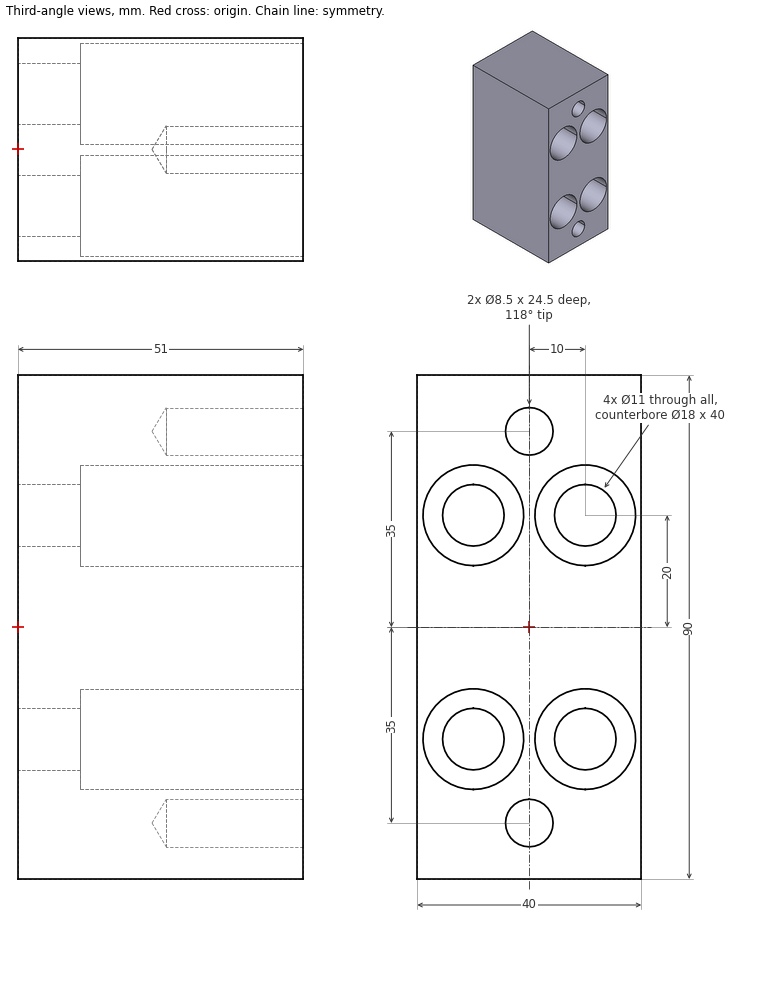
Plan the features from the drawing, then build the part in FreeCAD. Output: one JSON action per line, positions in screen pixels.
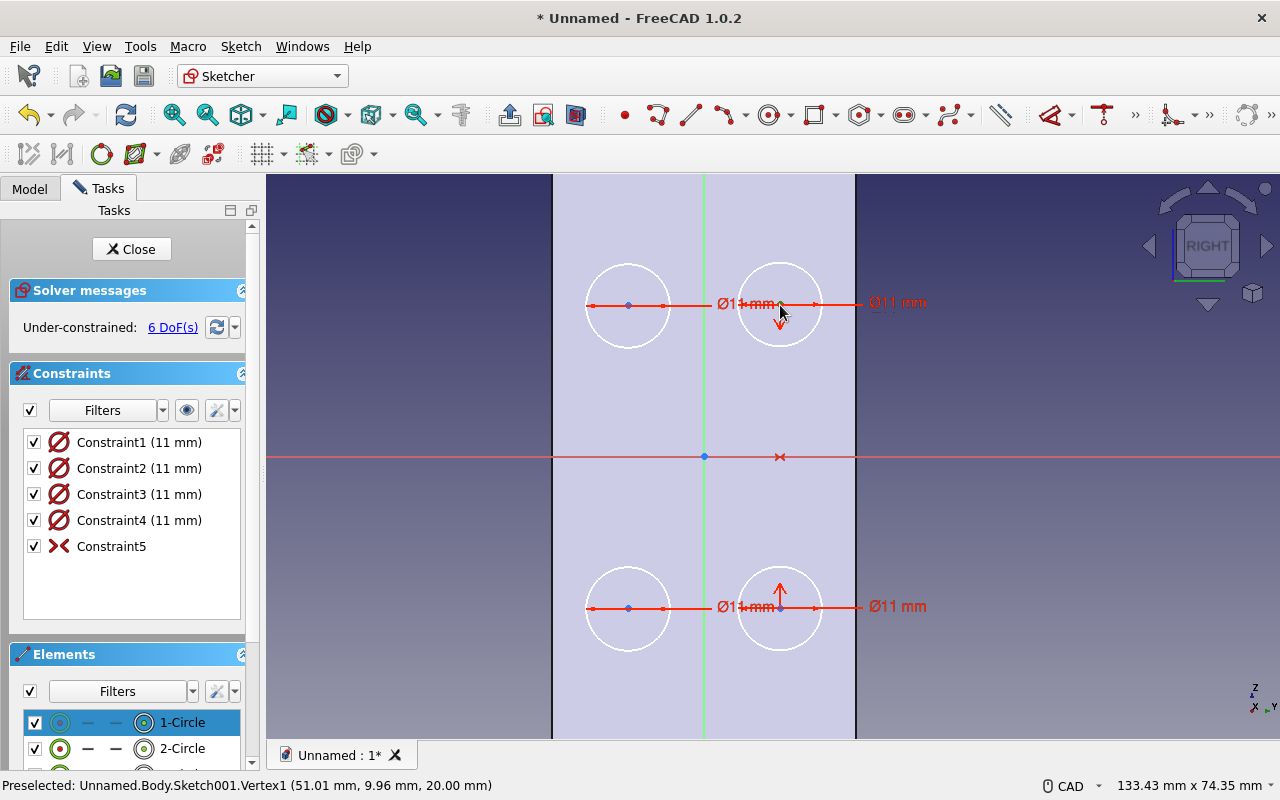
{"action": "left_click", "coordinate": [628, 306]}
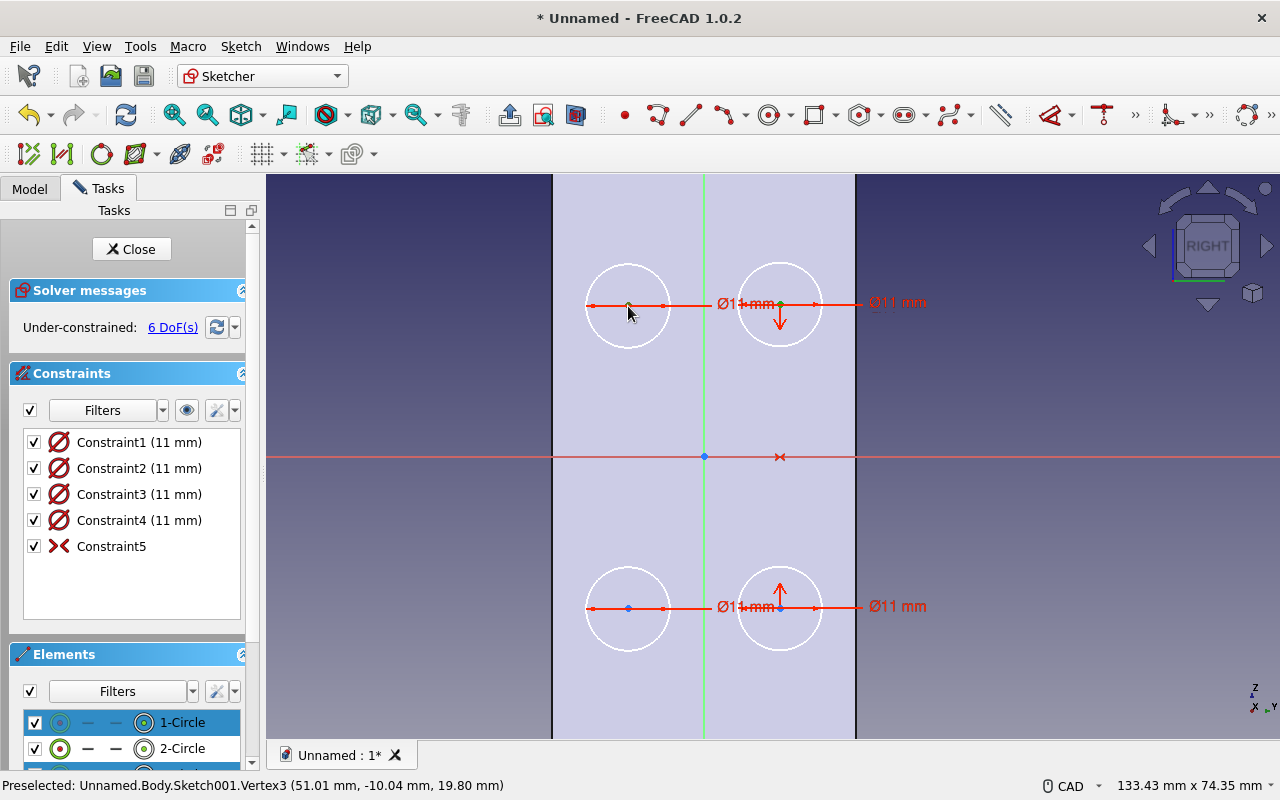
{"action": "left_click", "coordinate": [704, 675]}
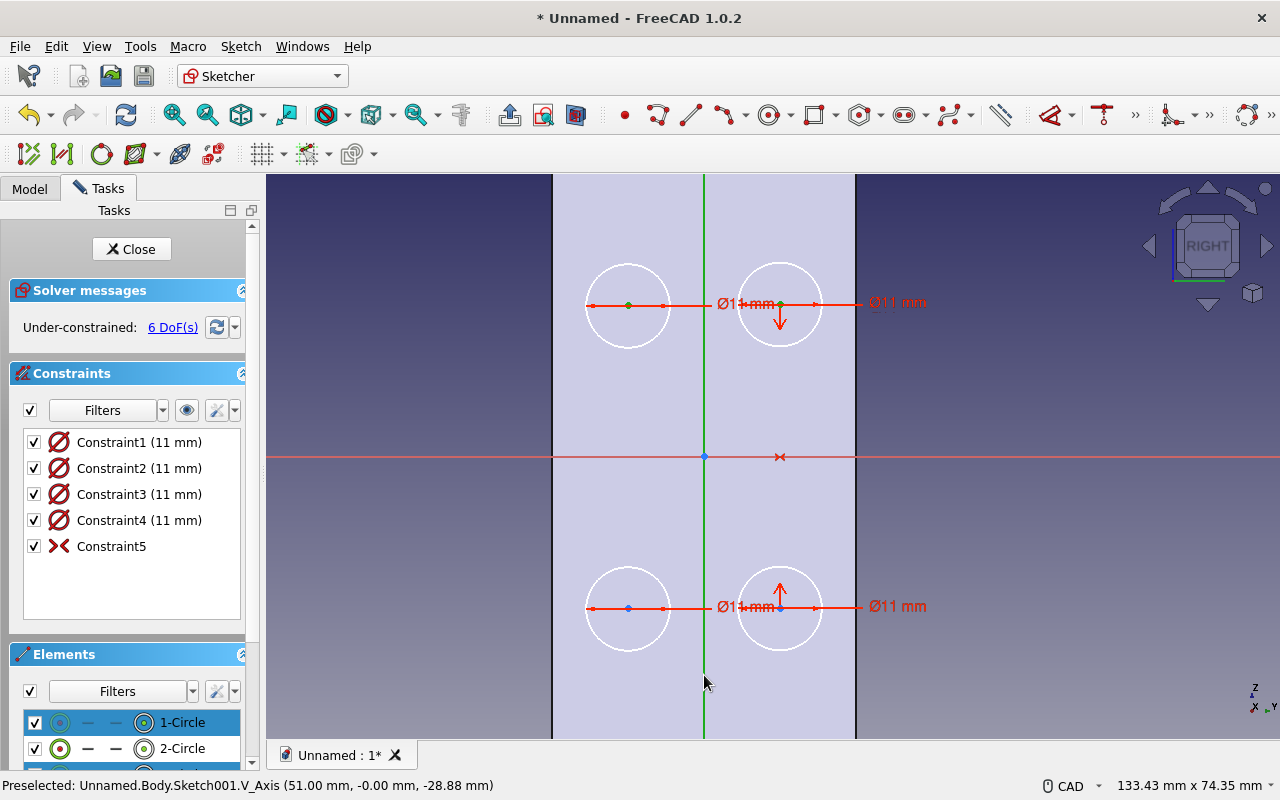
{"action": "key", "text": "s"}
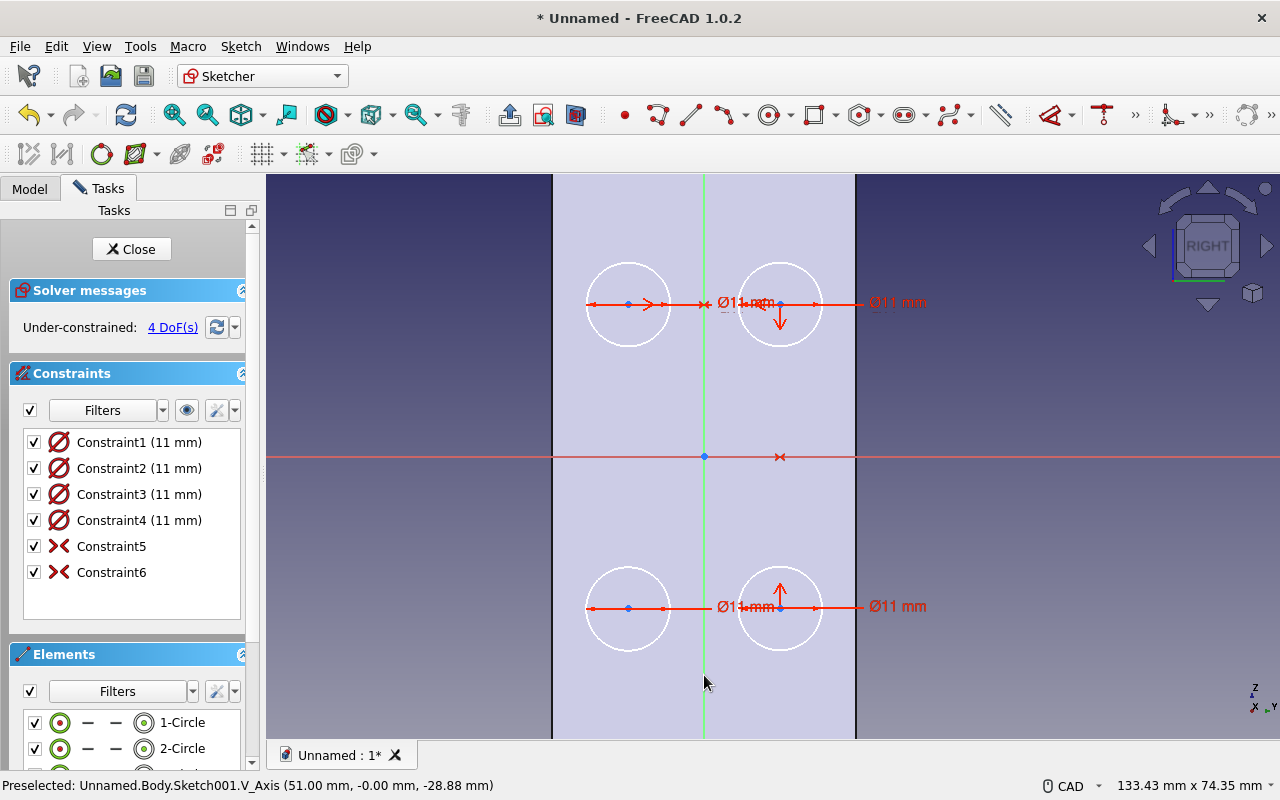
{"action": "left_click", "coordinate": [780, 608]}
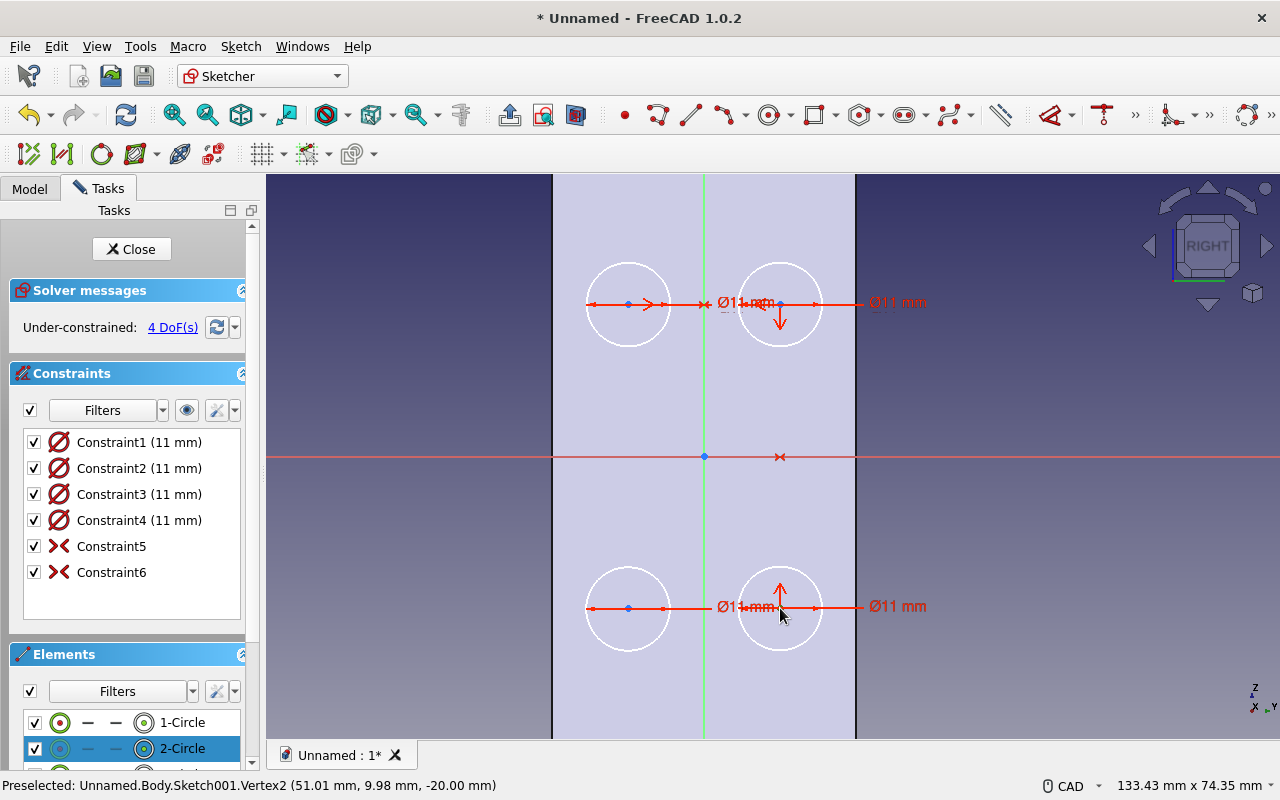
{"action": "left_click", "coordinate": [628, 609]}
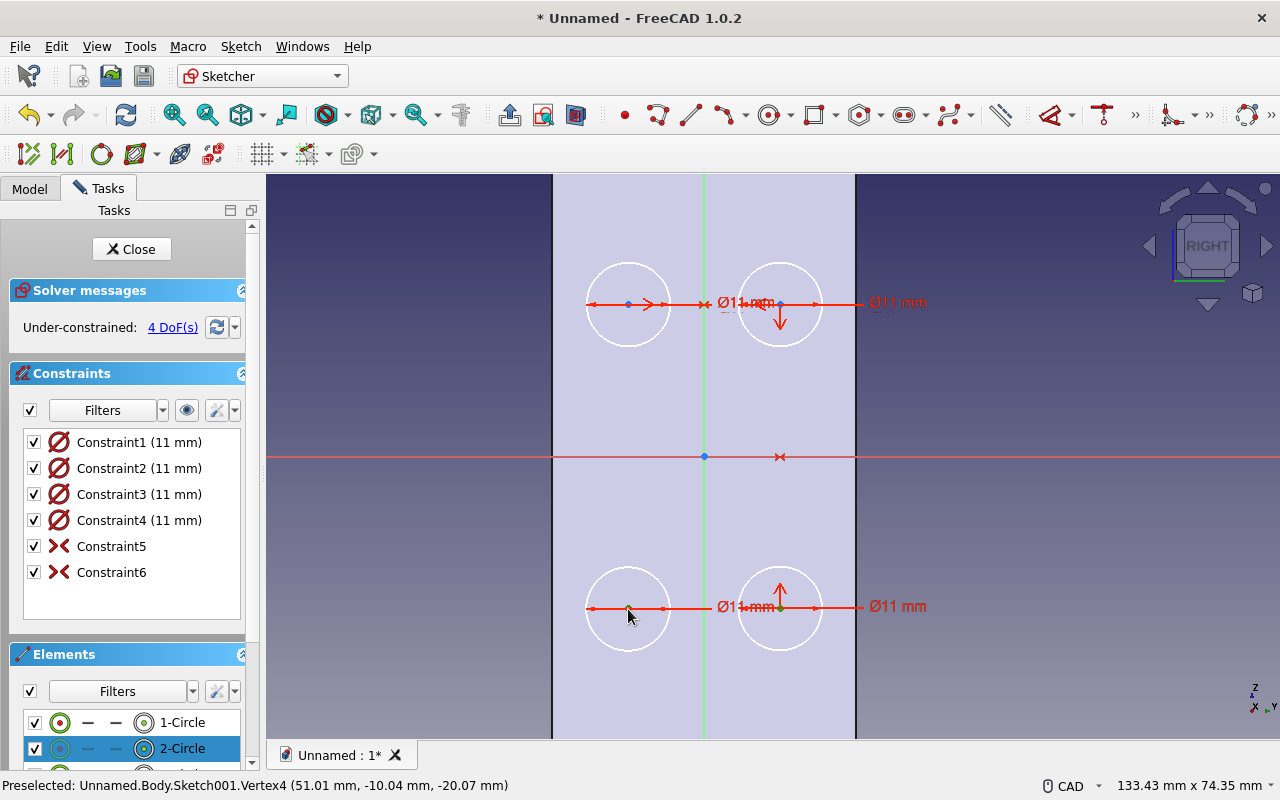
{"action": "left_click", "coordinate": [704, 675]}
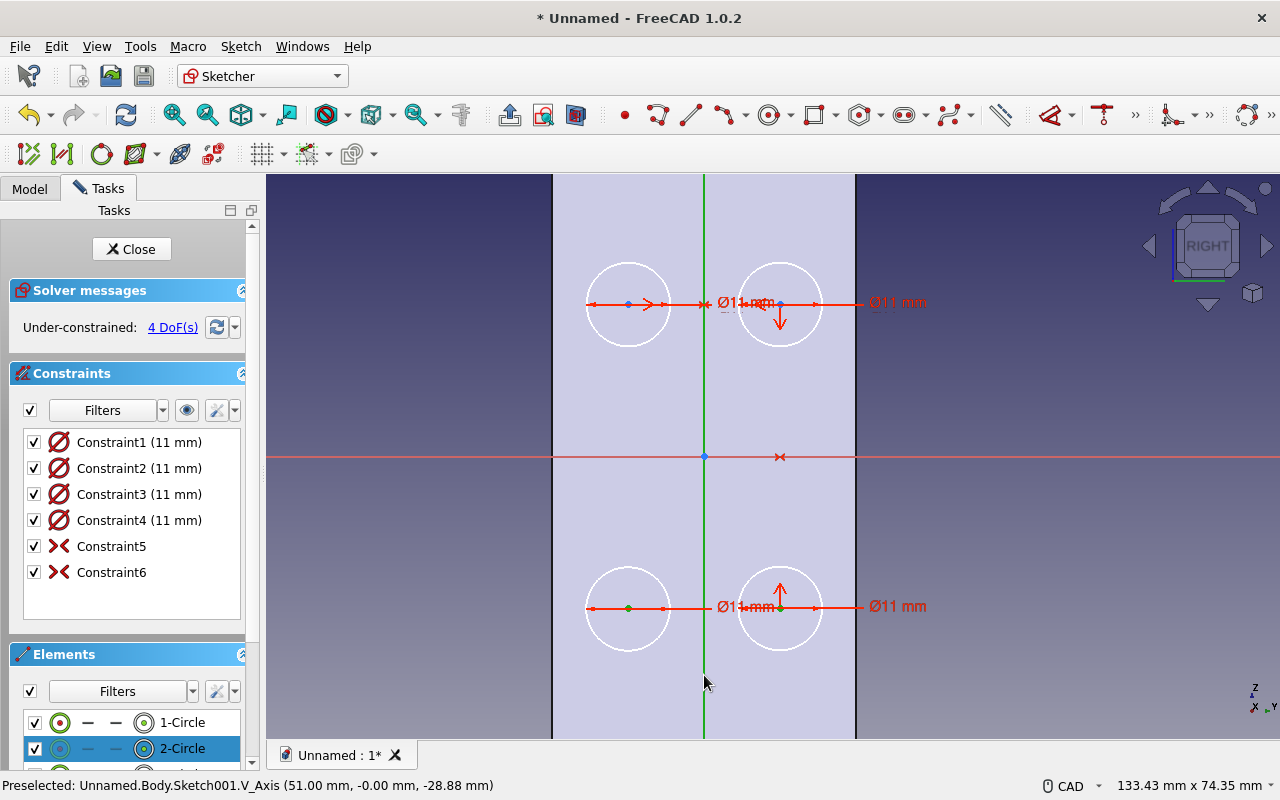
{"action": "key", "text": "s"}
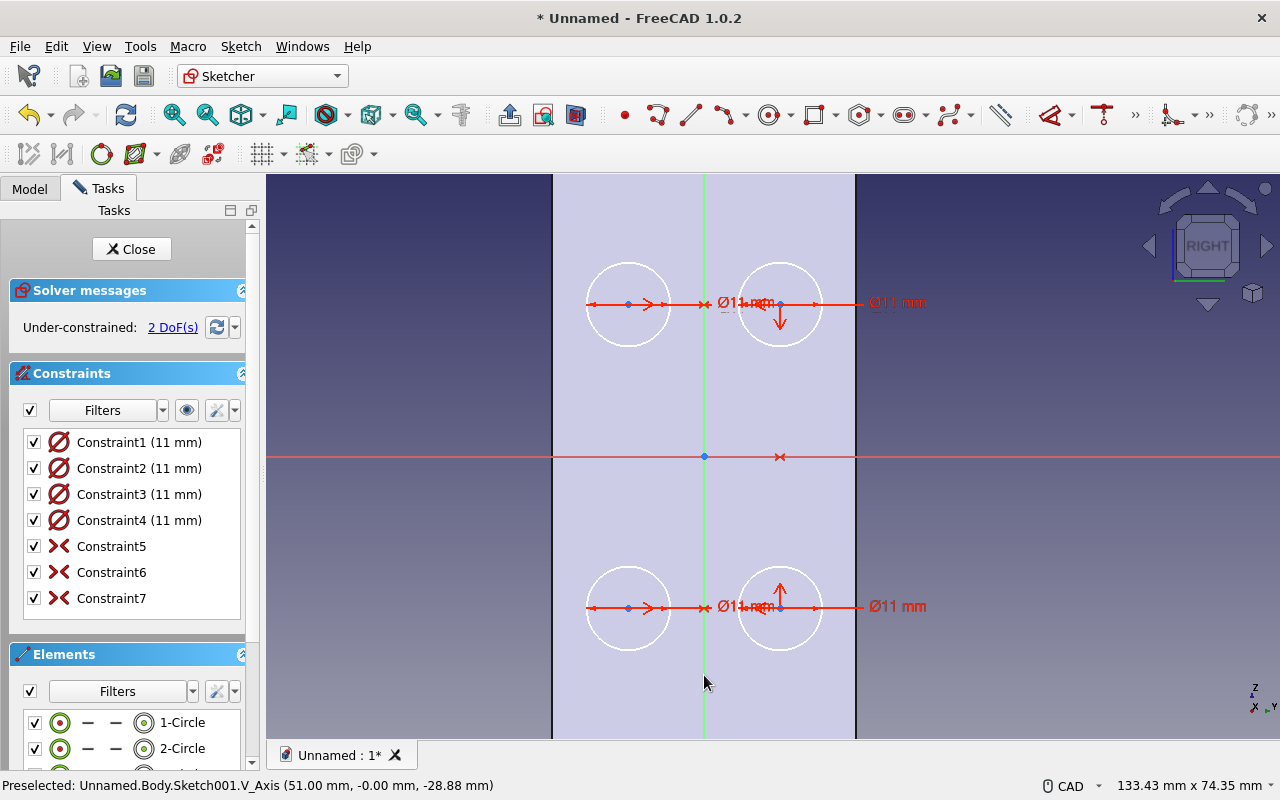
{"action": "left_click", "coordinate": [1050, 116]}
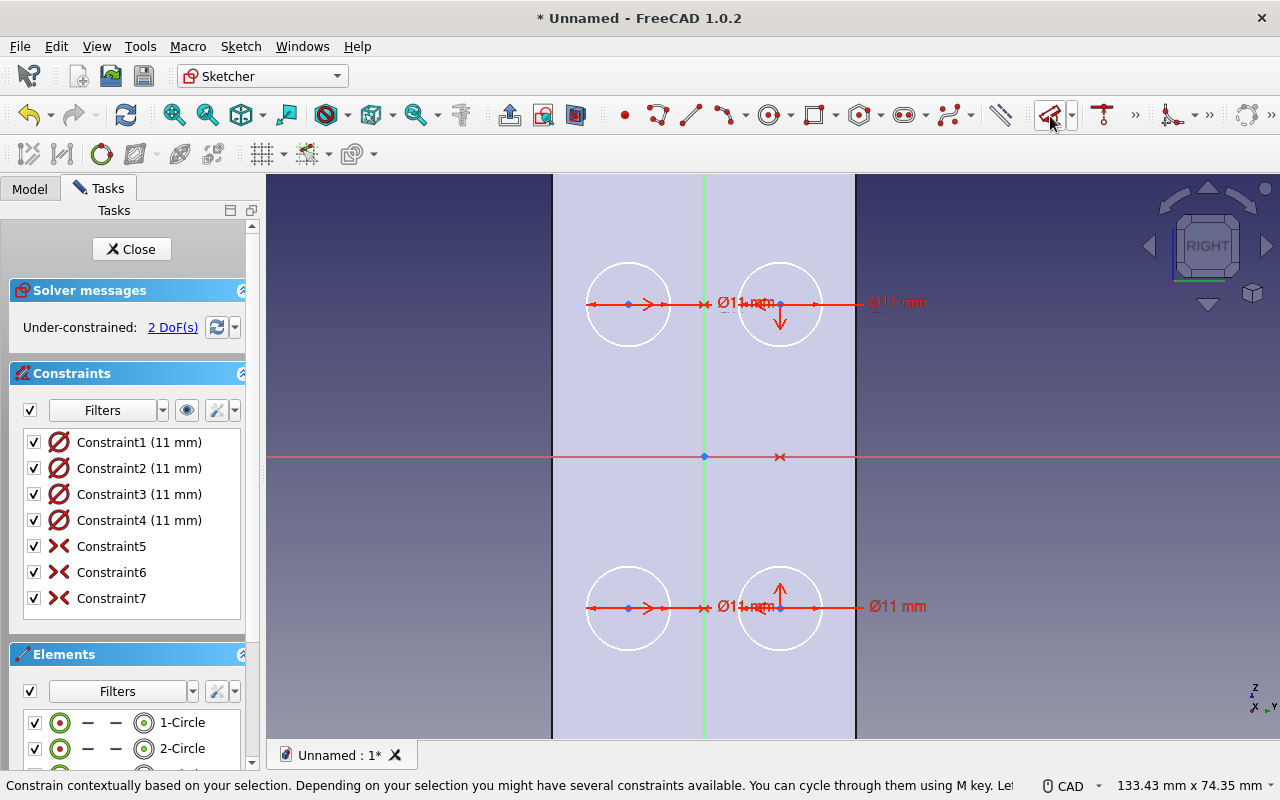
{"action": "left_click", "coordinate": [780, 305]}
{"action": "left_click", "coordinate": [725, 271]}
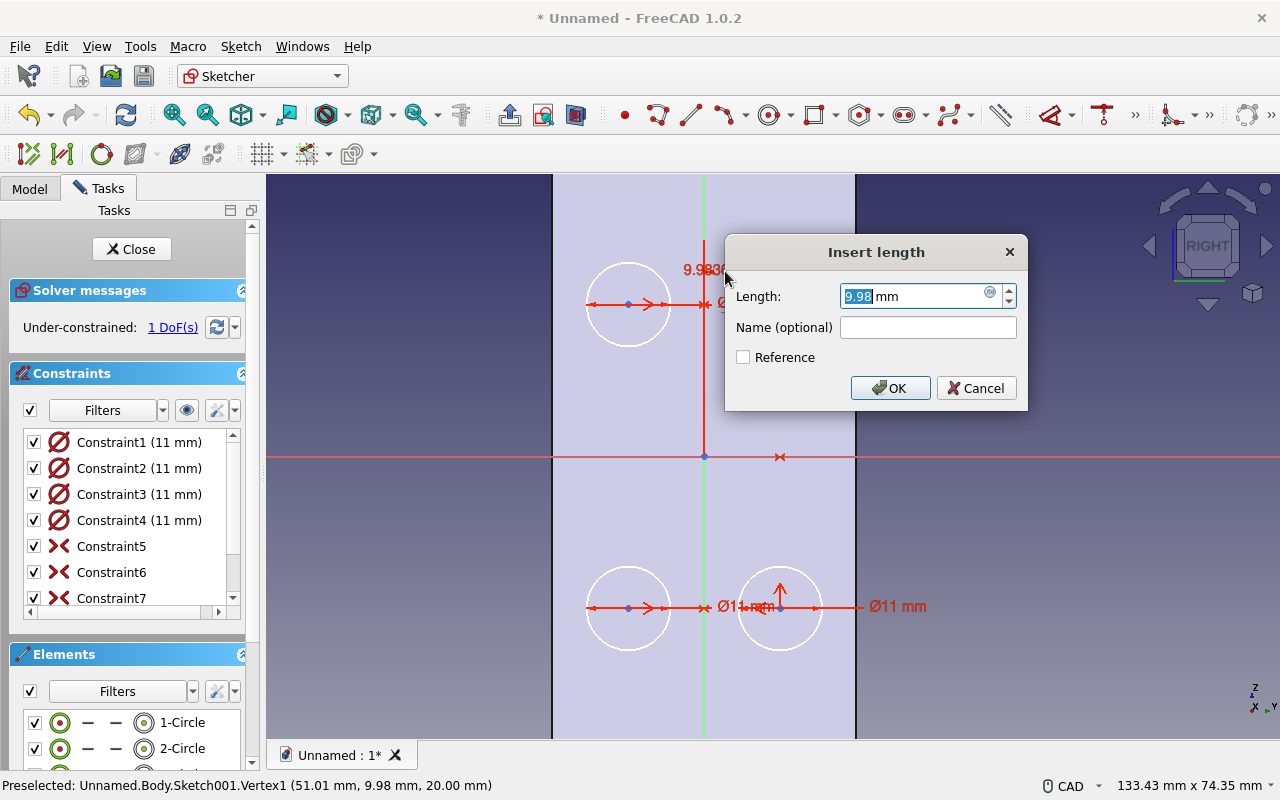
{"action": "type", "text": "10"}
{"action": "key", "text": "Return"}